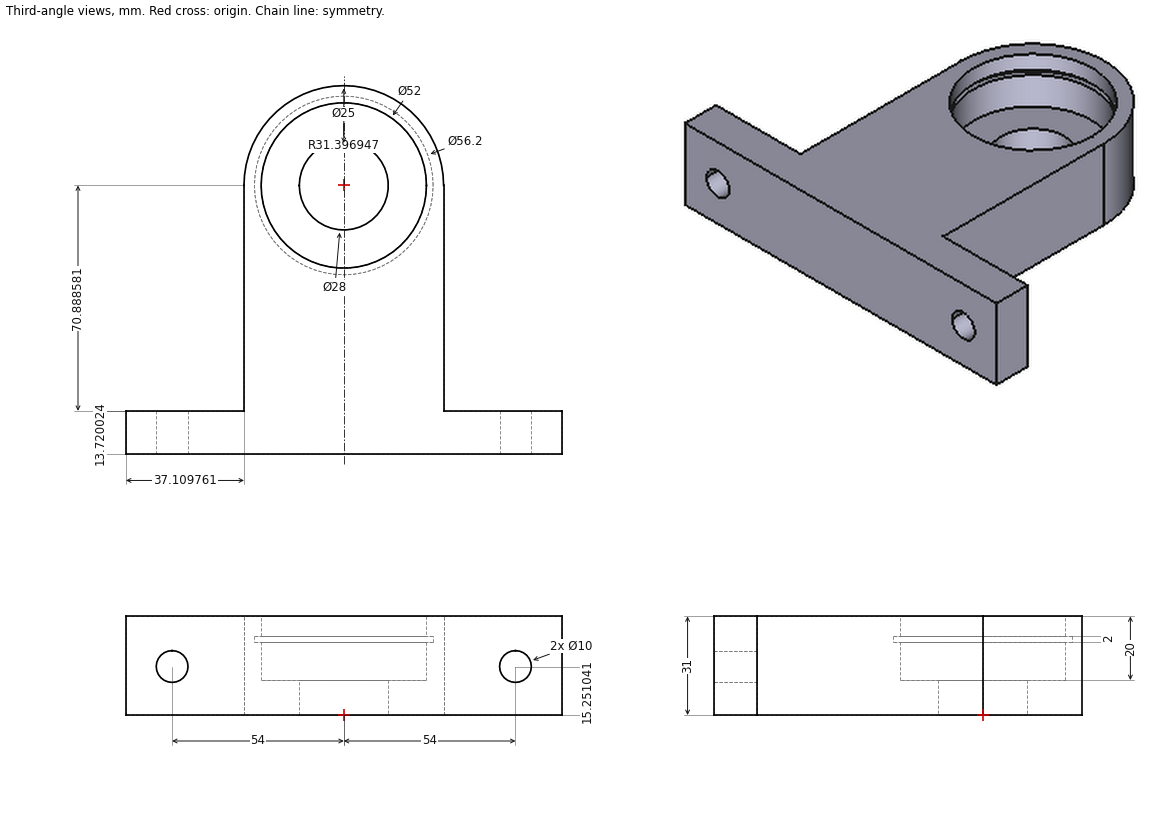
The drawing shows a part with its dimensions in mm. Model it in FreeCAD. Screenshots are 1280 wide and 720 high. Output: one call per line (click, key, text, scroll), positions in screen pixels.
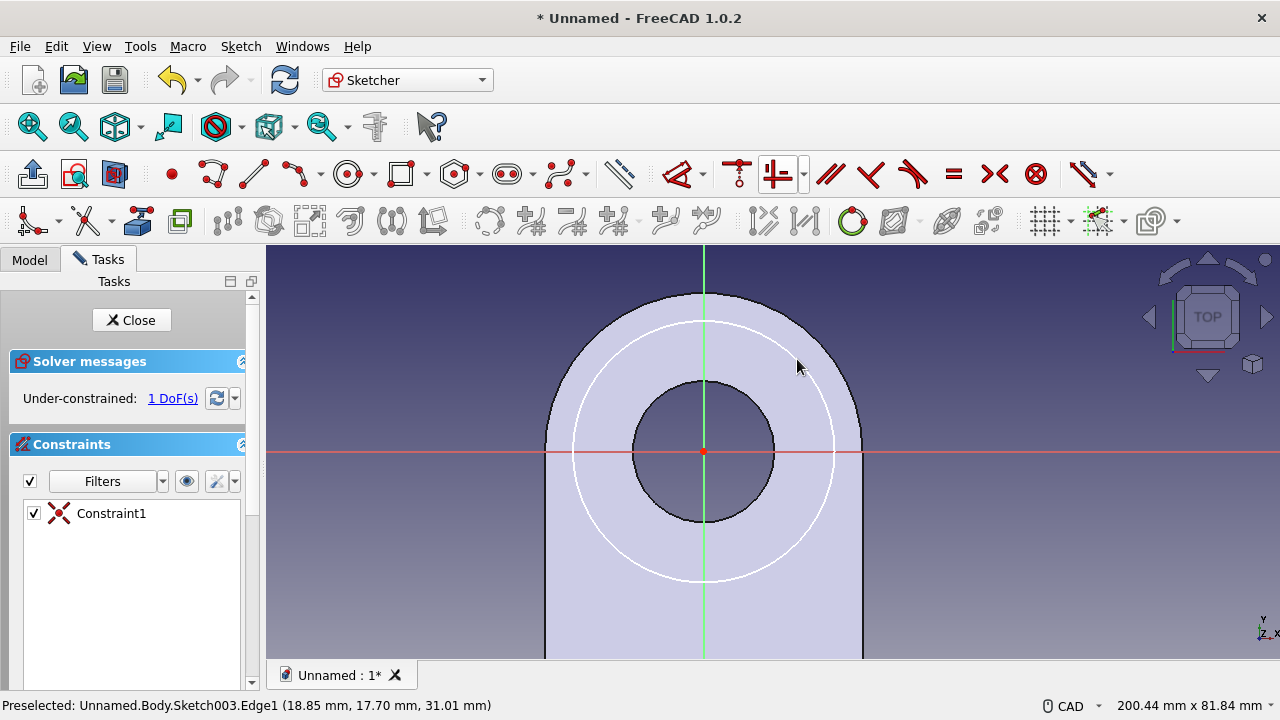
click(676, 174)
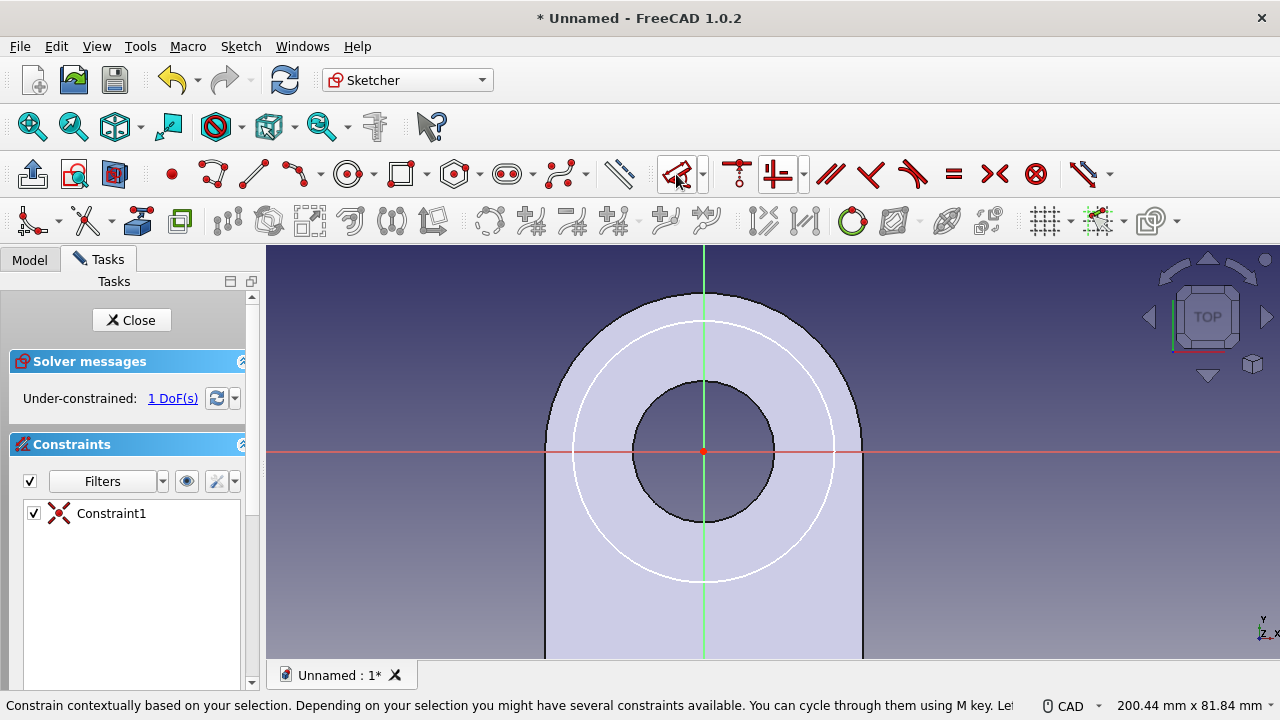
click(796, 359)
click(819, 336)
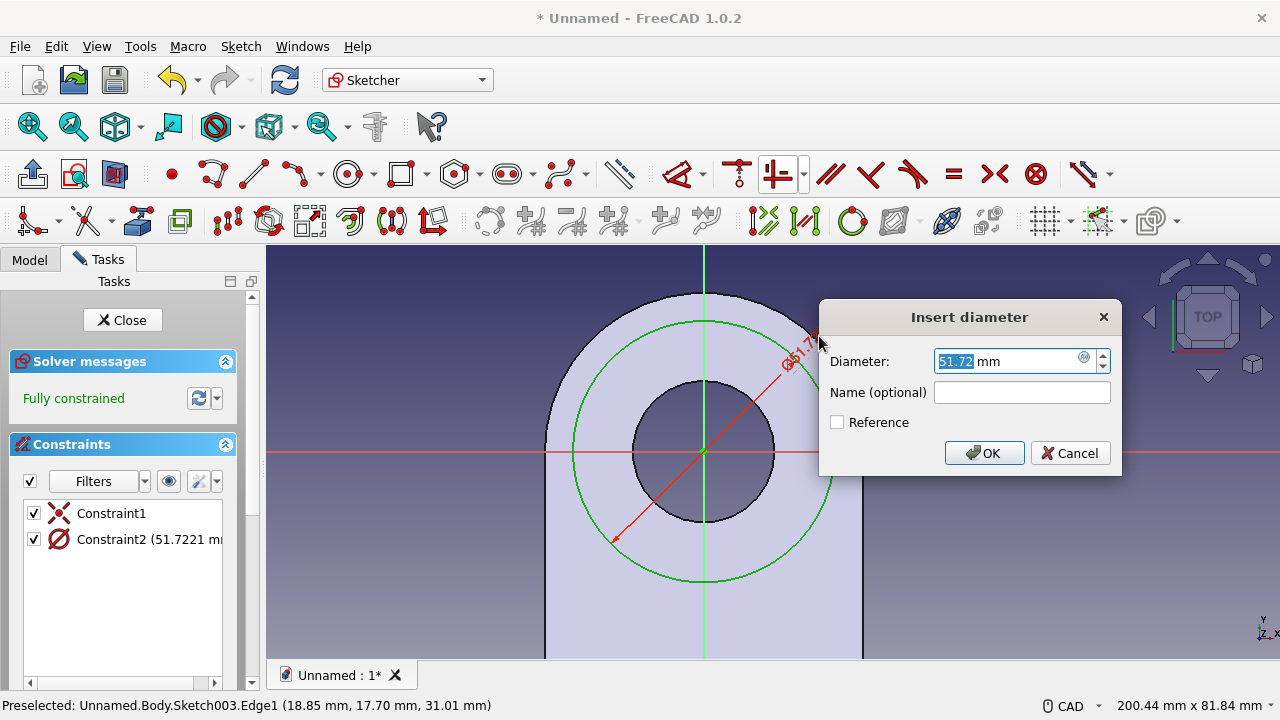
text(52)
key(Return)
key(Escape)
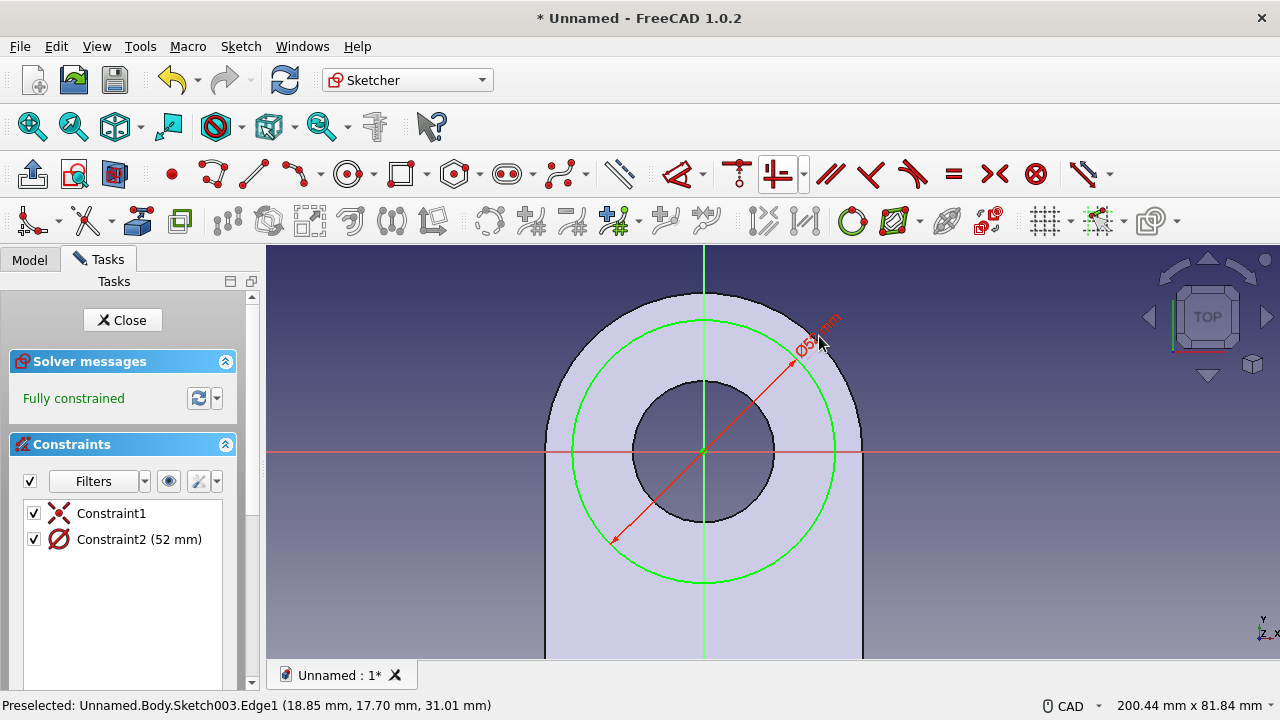
click(123, 320)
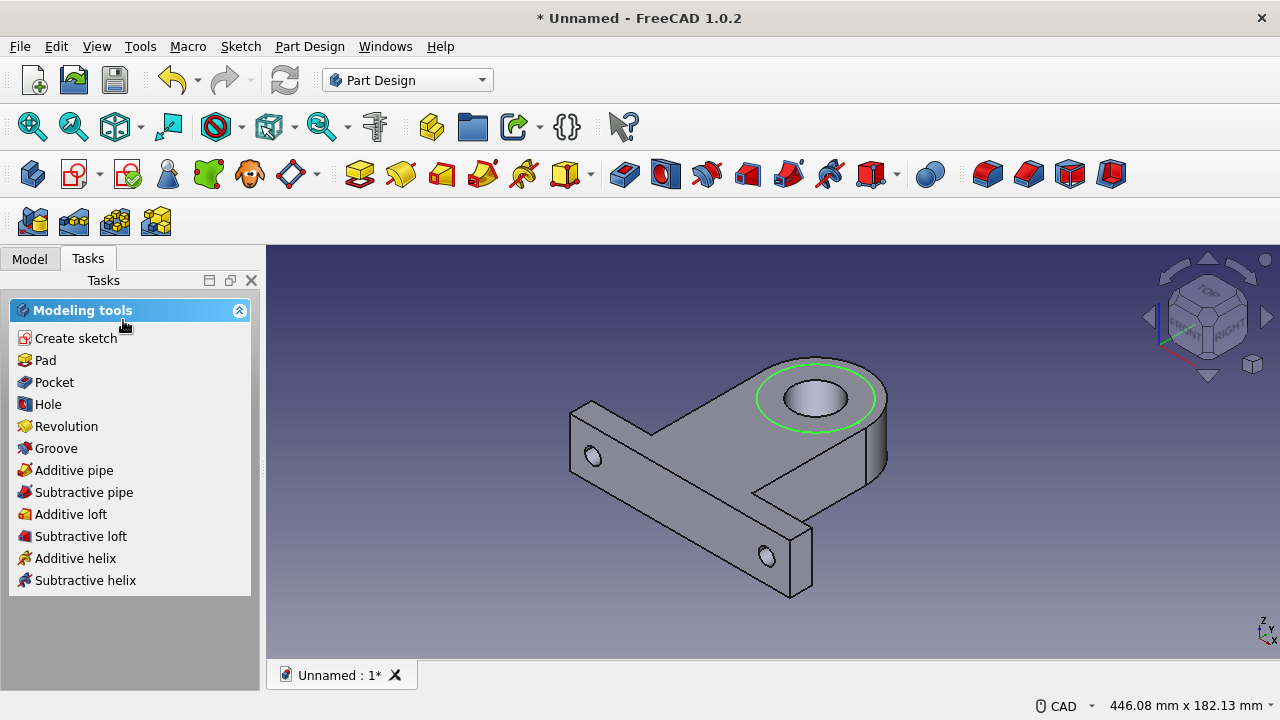
click(625, 174)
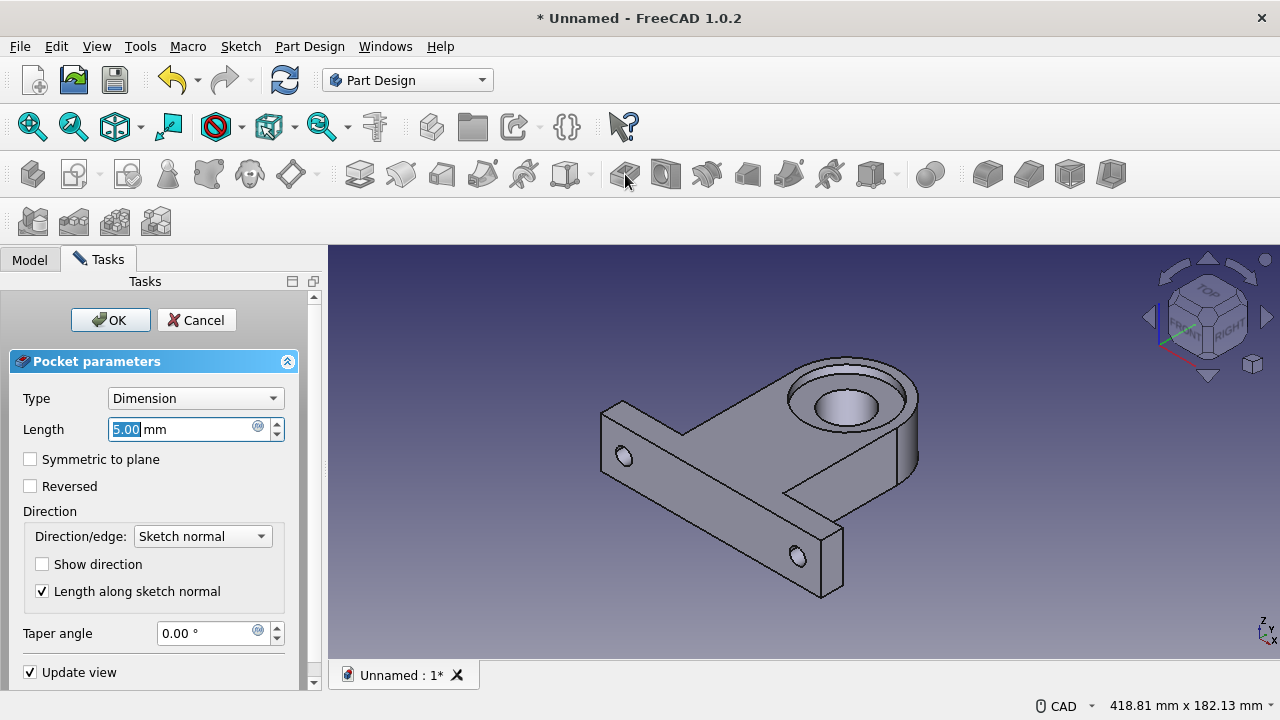
text(20)
key(Tab)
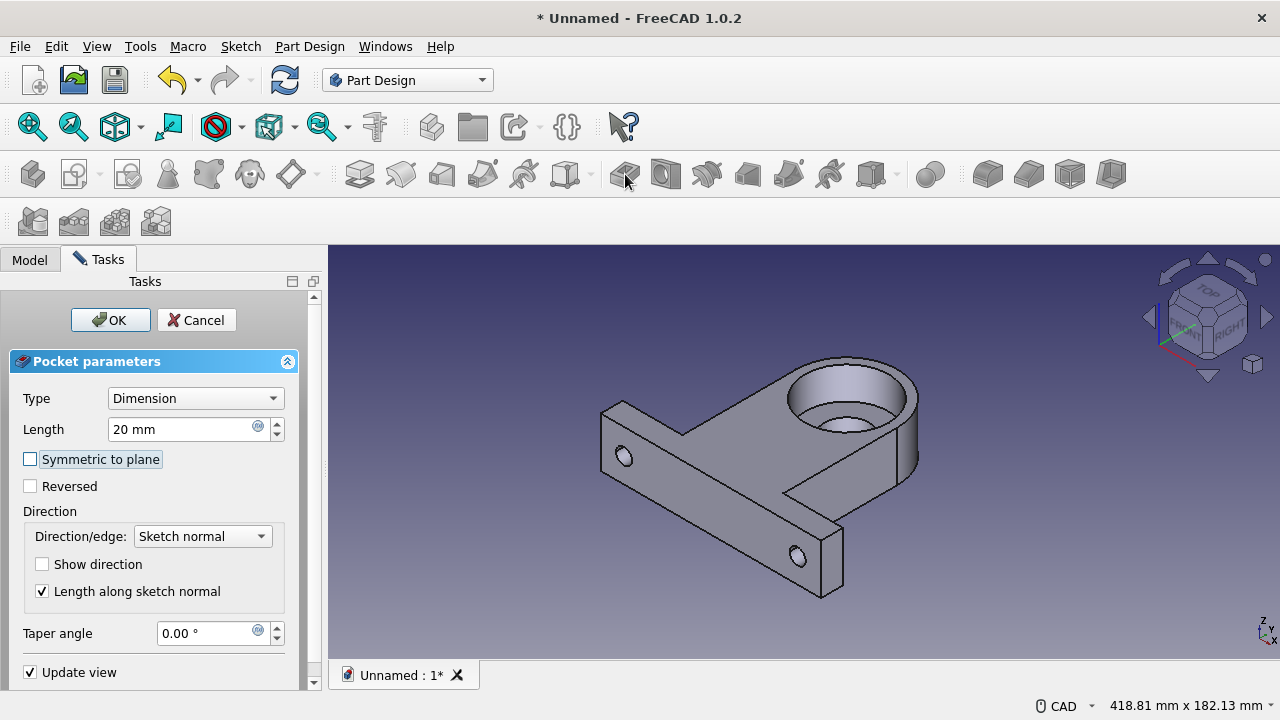
click(111, 320)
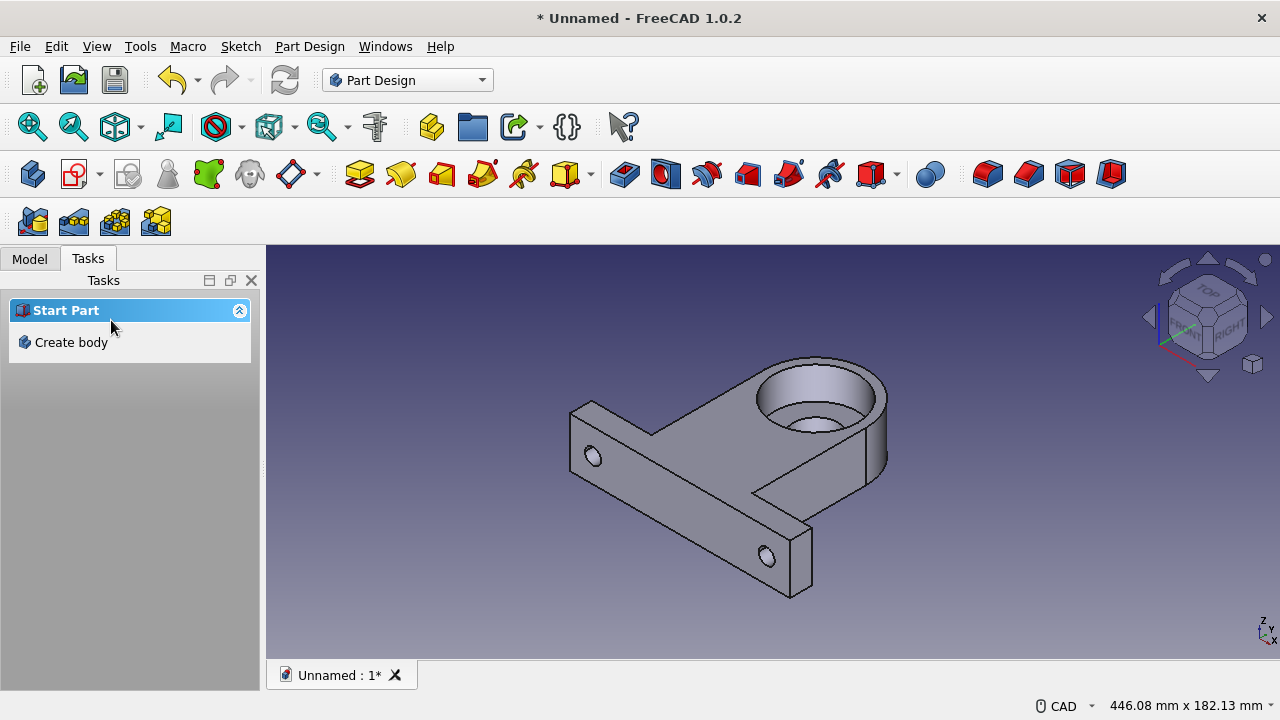
click(30, 258)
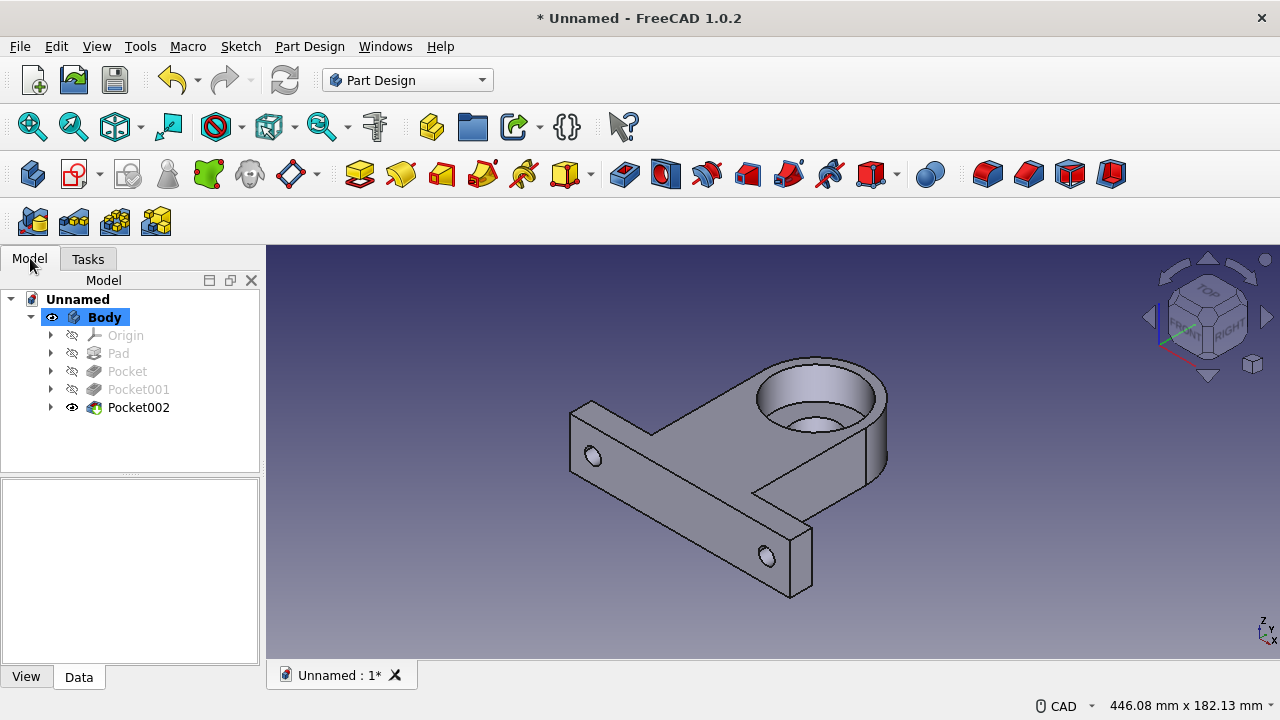
click(51, 335)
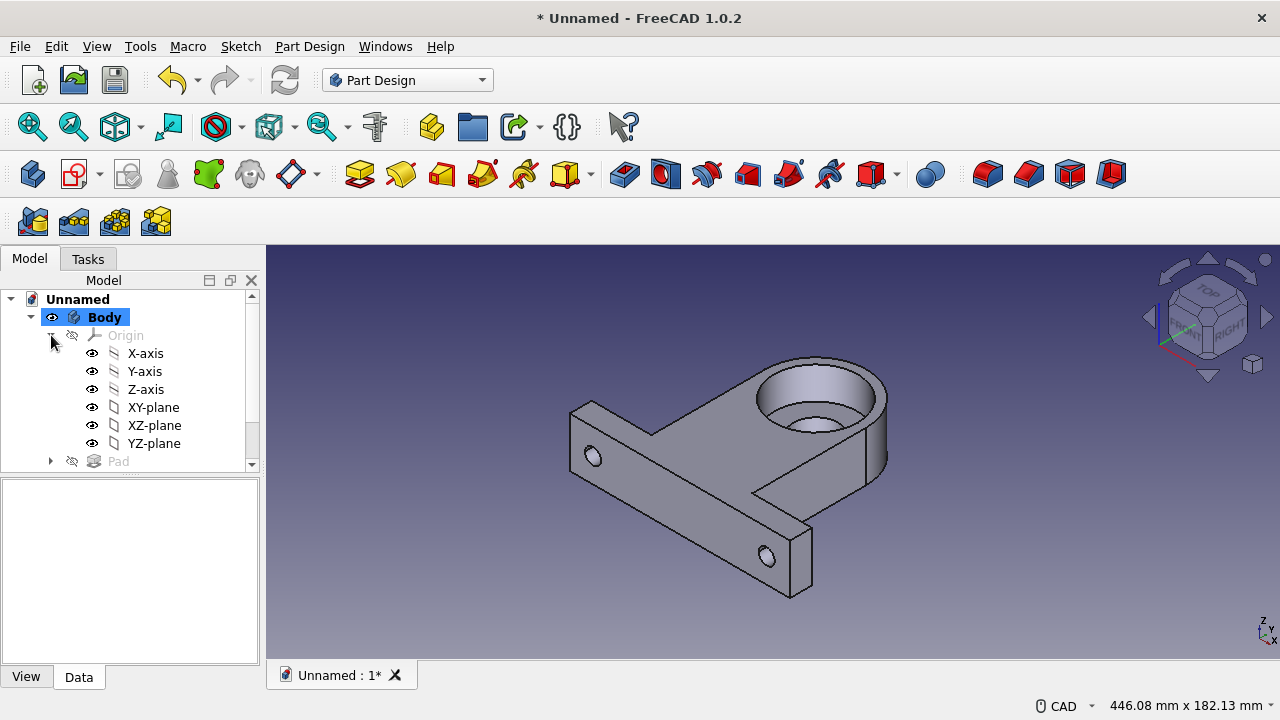
click(137, 407)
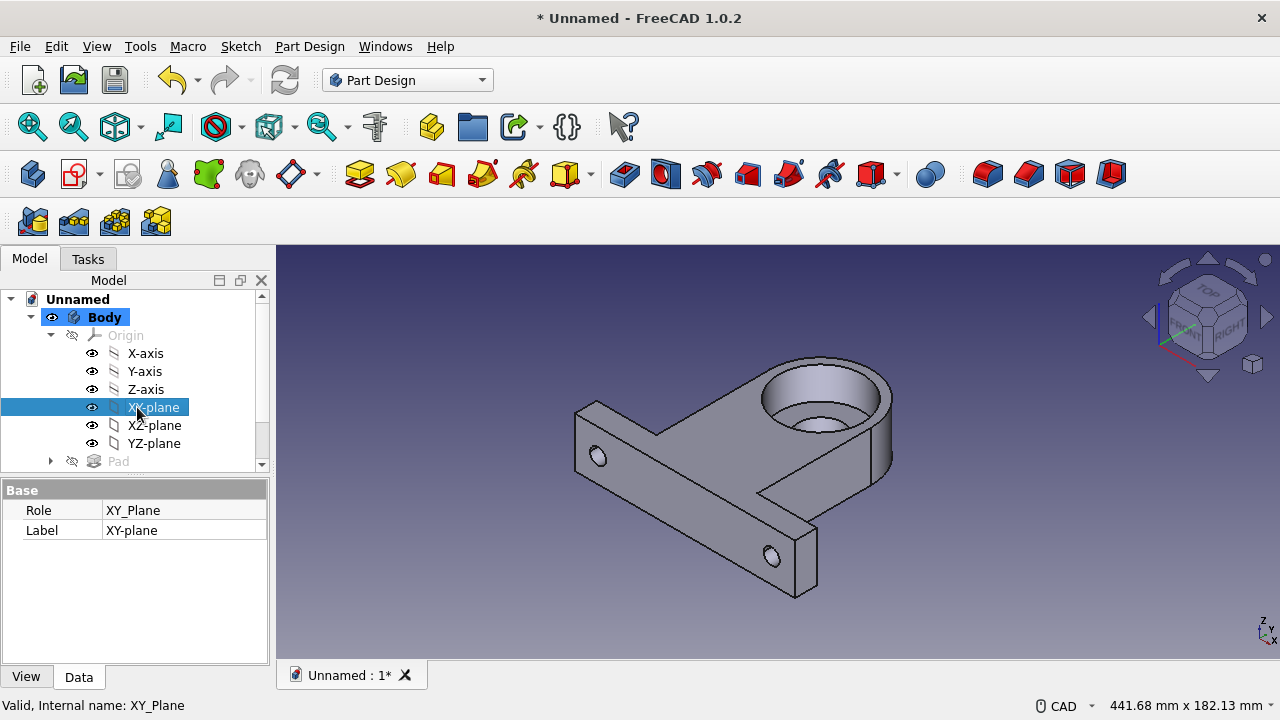
click(290, 174)